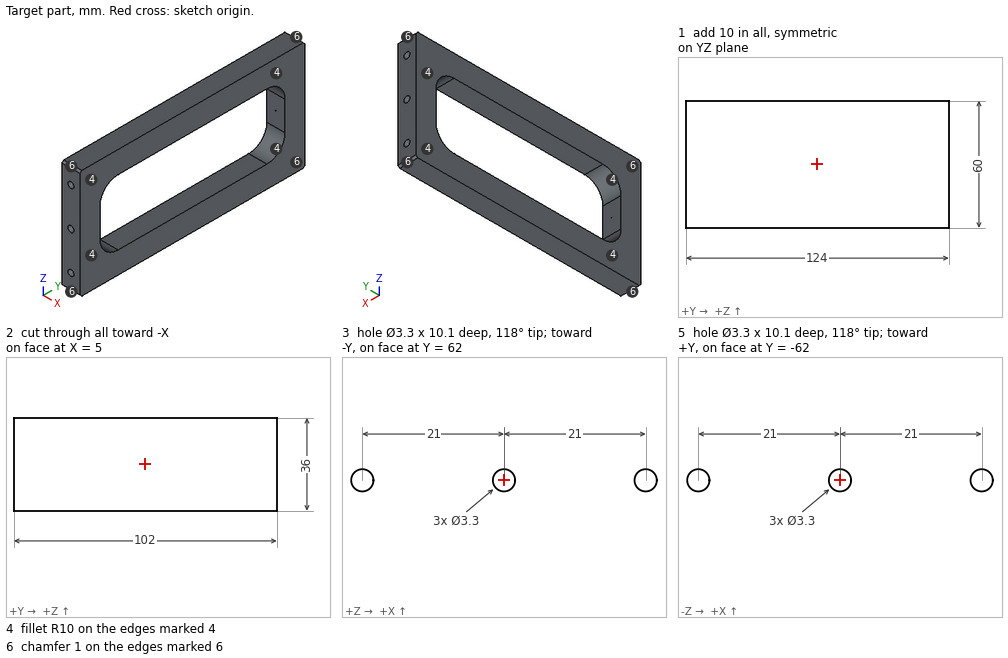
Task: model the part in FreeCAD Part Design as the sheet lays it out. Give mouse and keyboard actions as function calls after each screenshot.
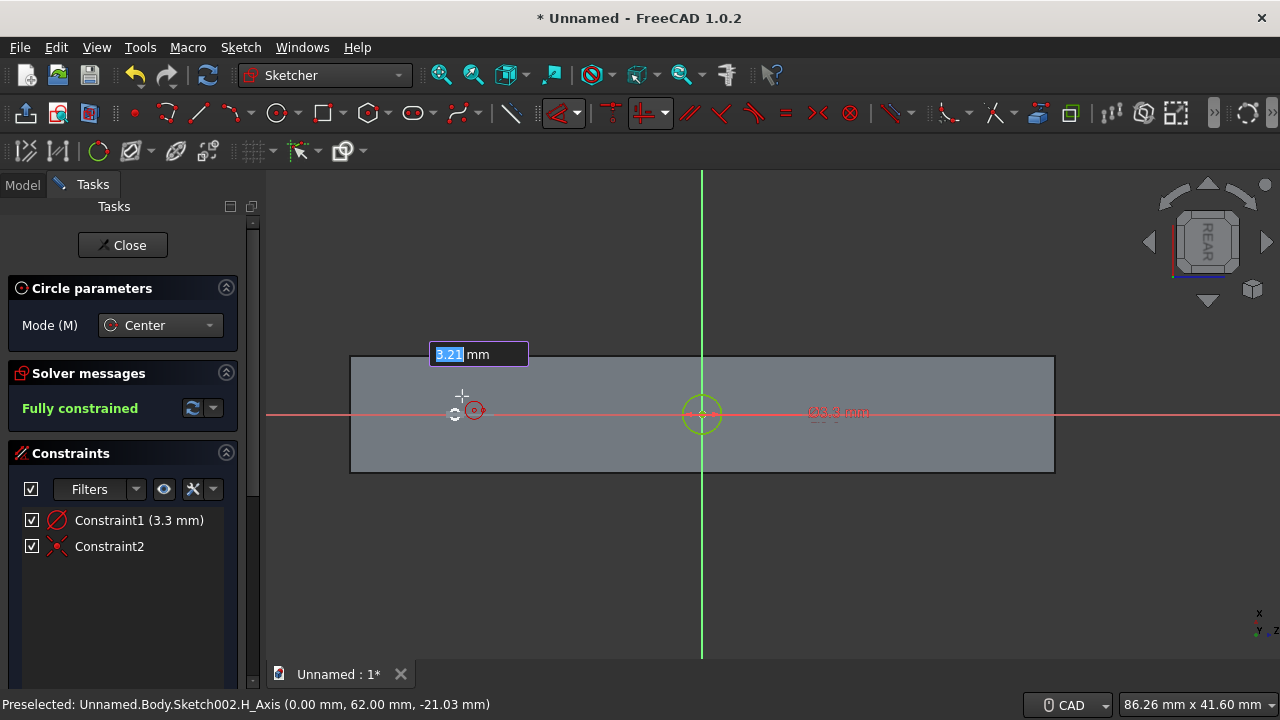
text(3.3)
key(Return)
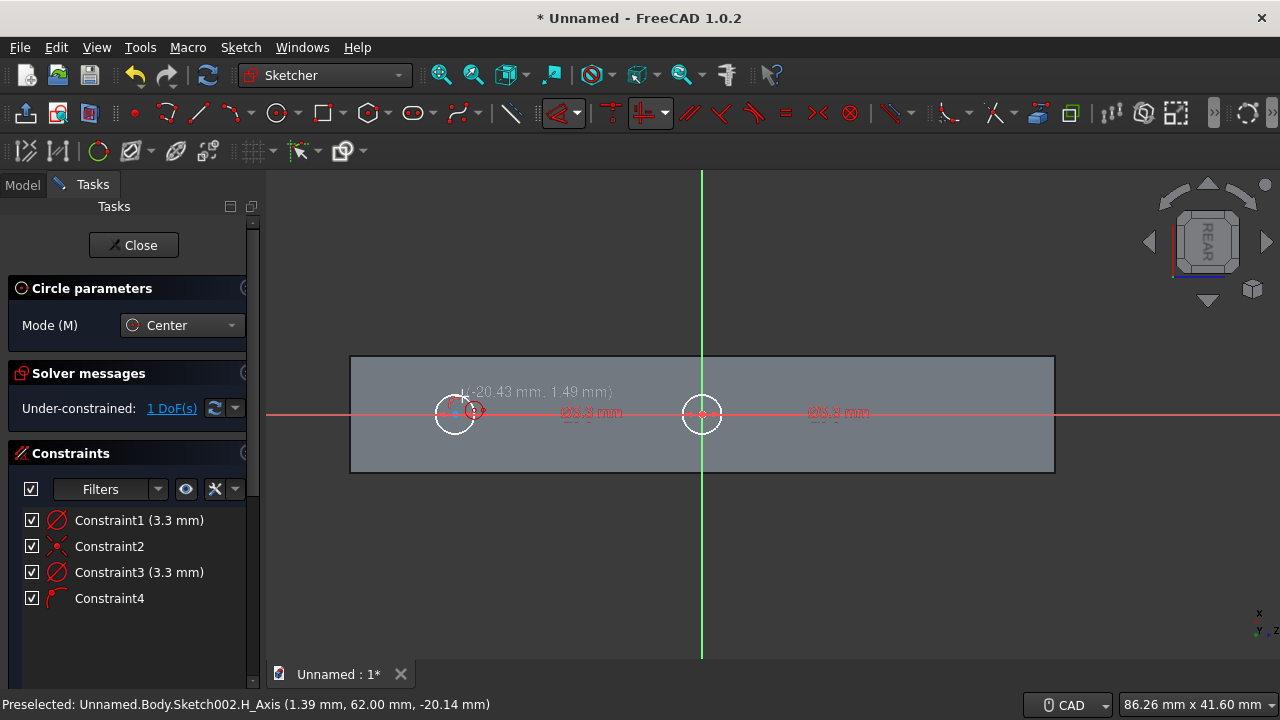
click(949, 414)
move(956, 396)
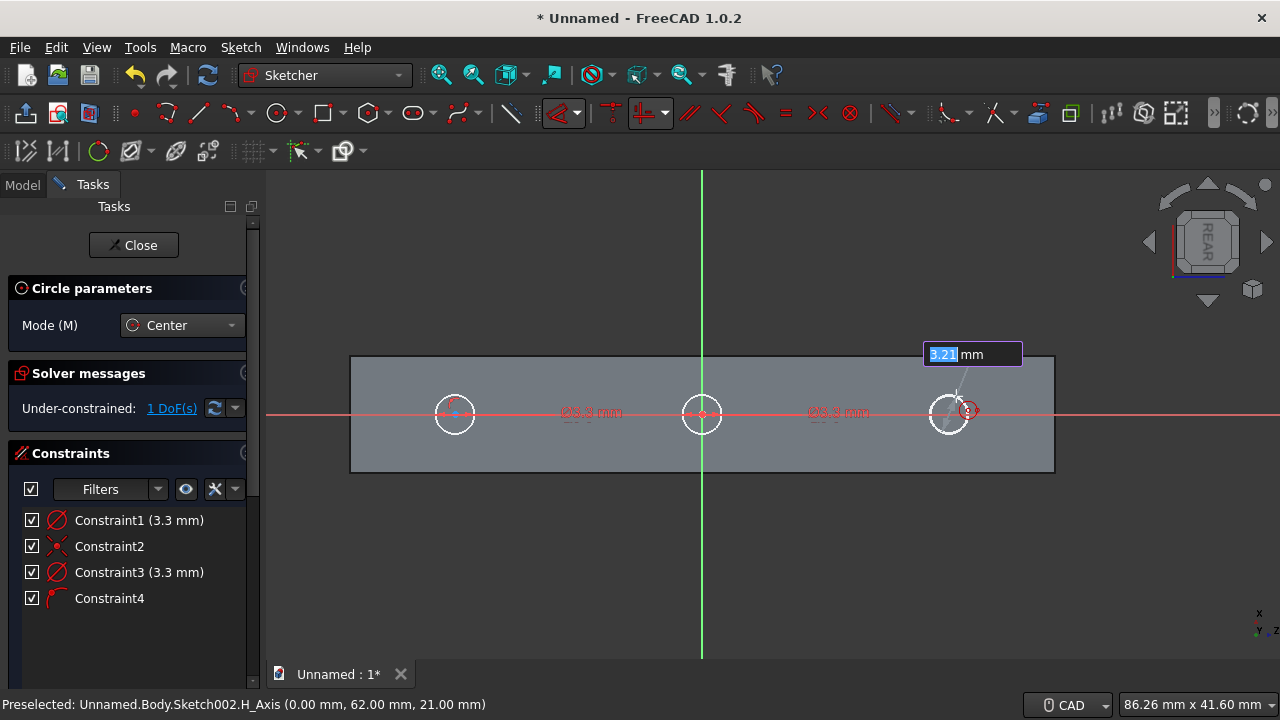
text(3.3)
key(Return)
key(Escape)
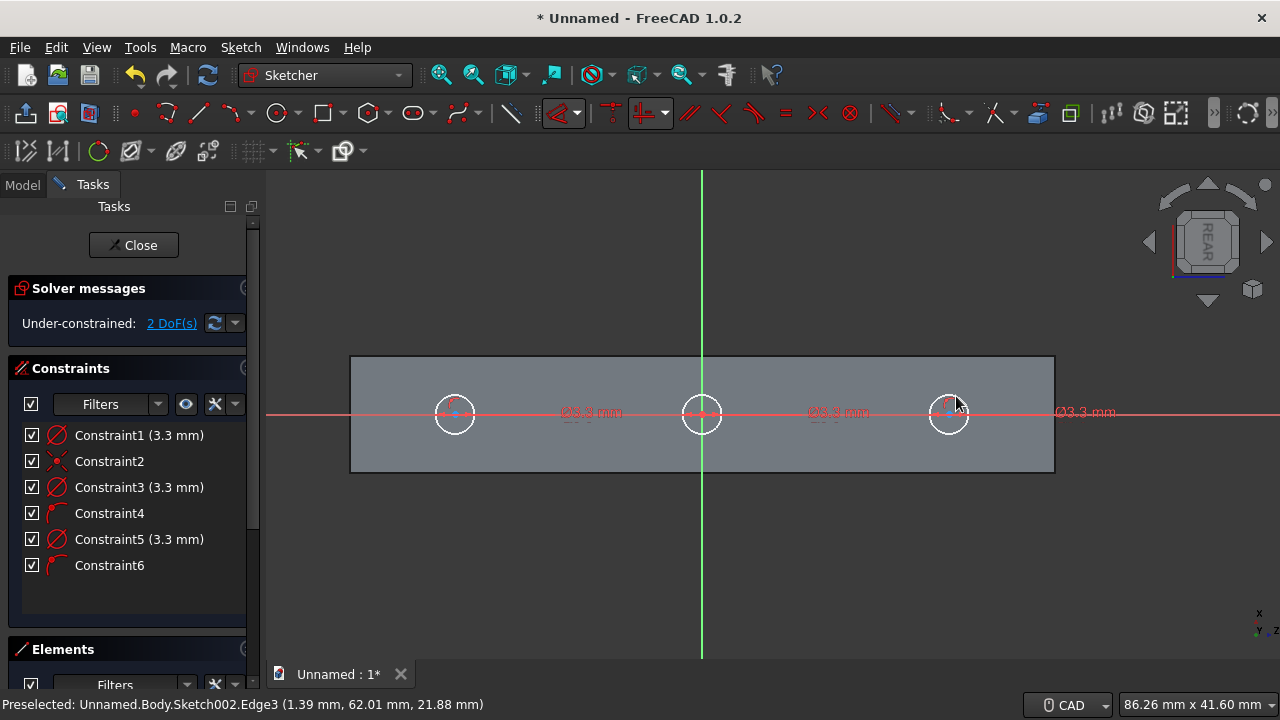
click(455, 414)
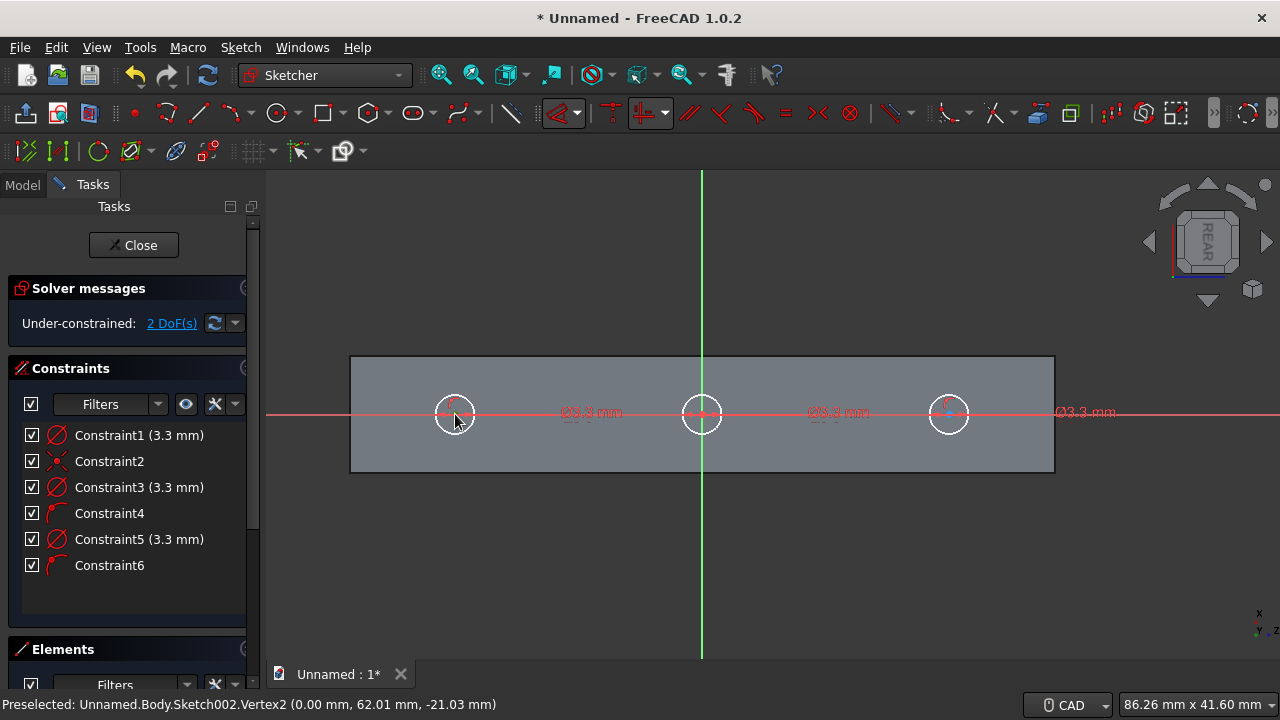
click(580, 114)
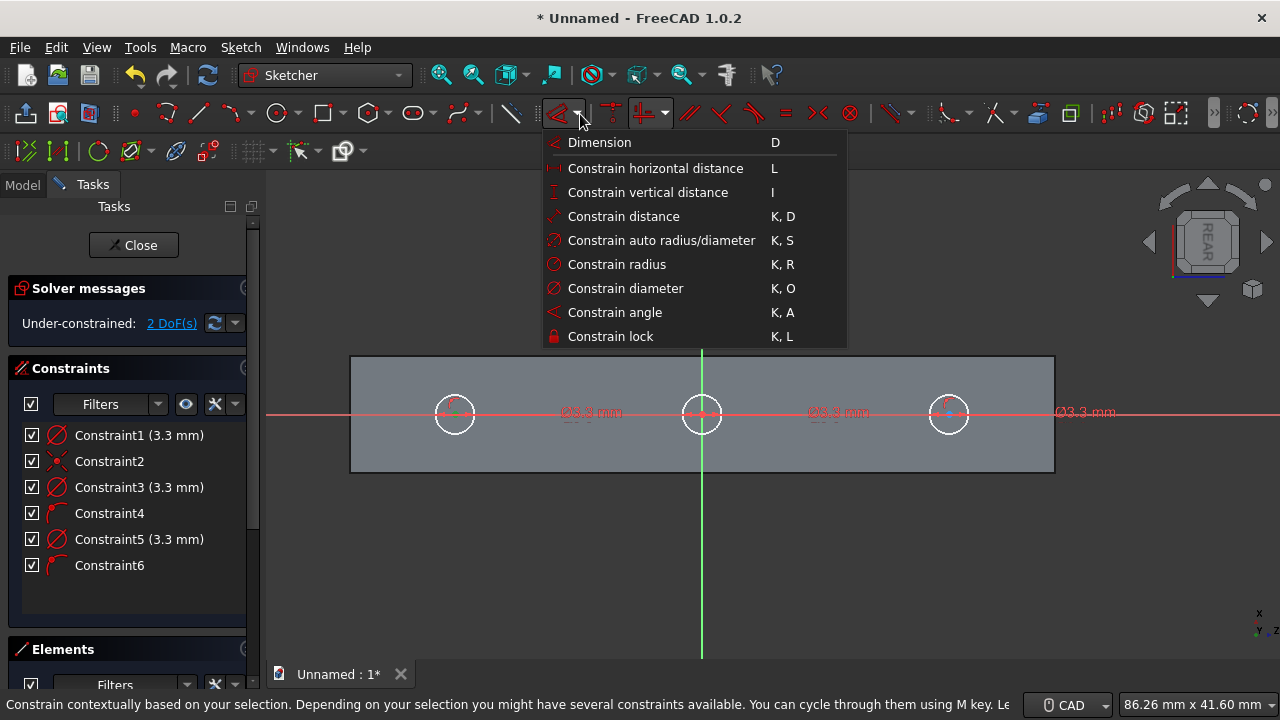
click(695, 168)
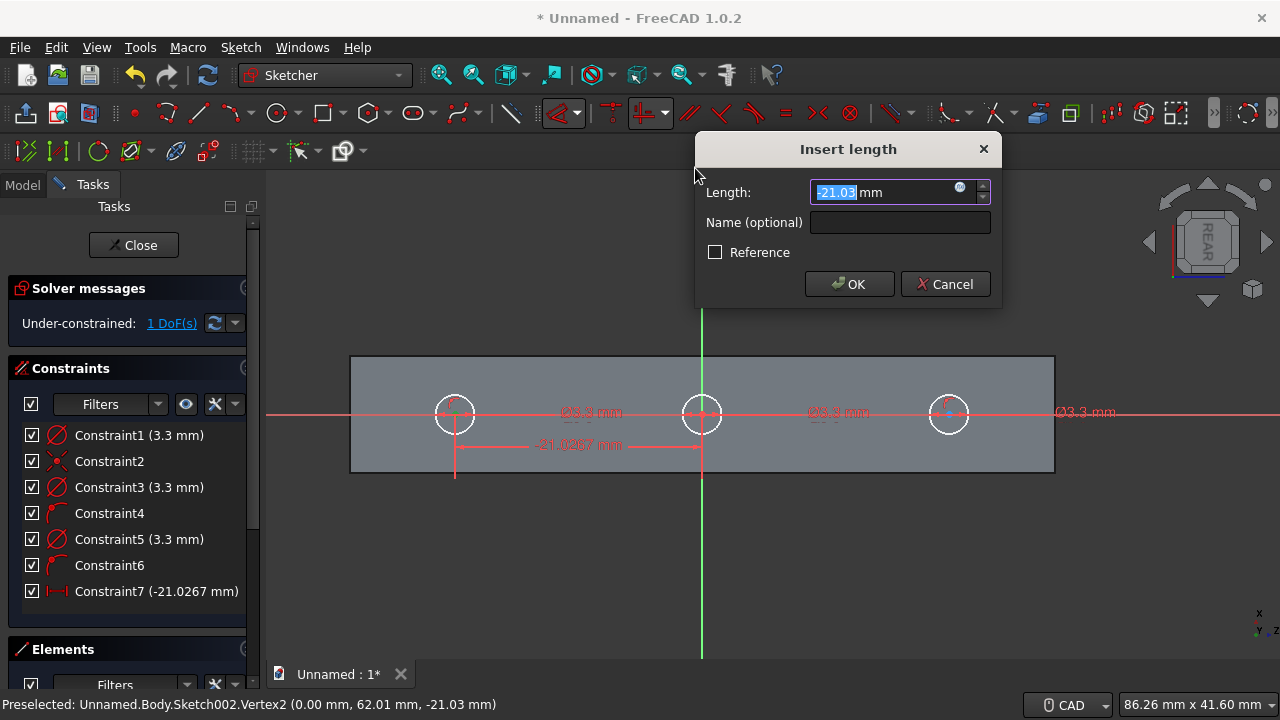
text(-21)
key(Return)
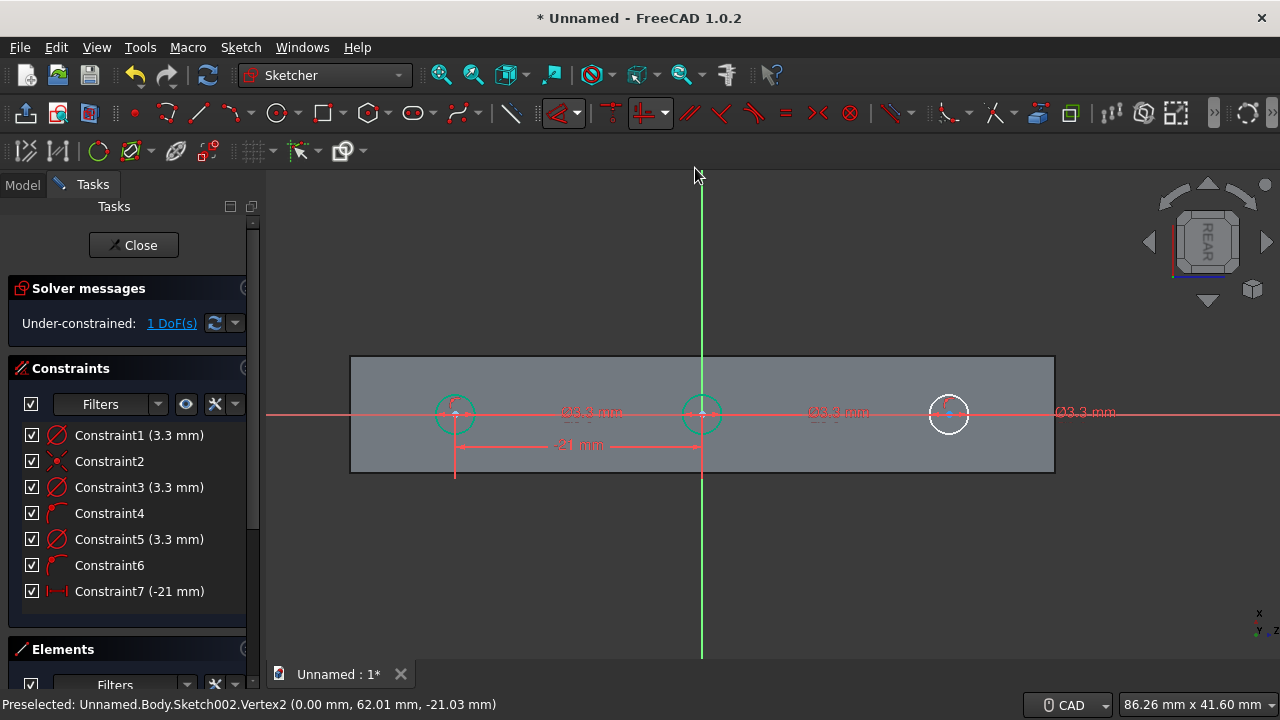
click(949, 414)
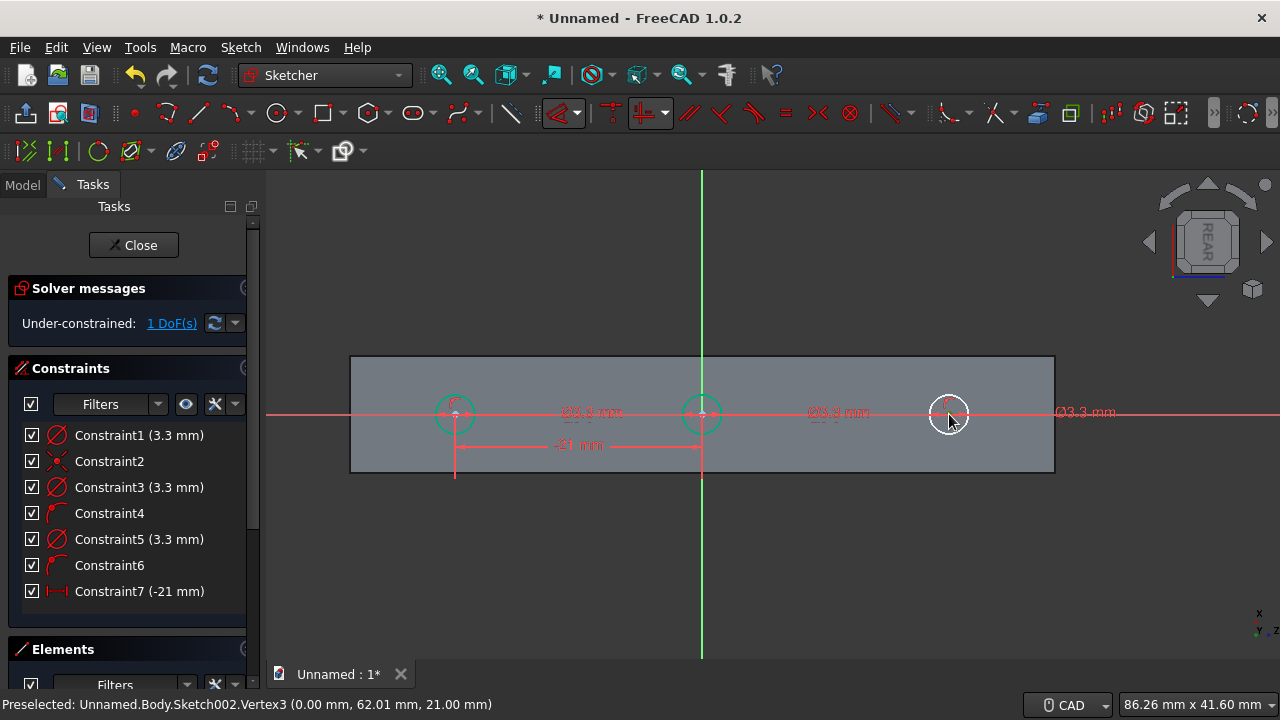
key(l)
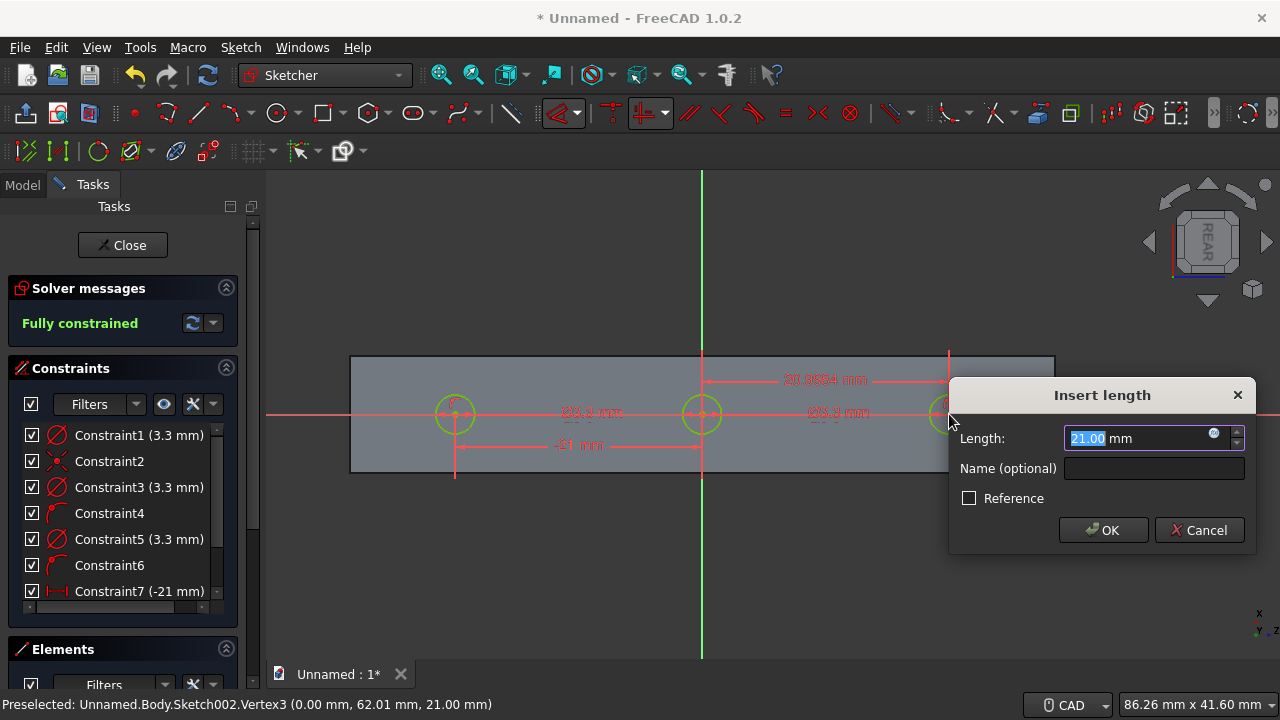
text(21)
key(Return)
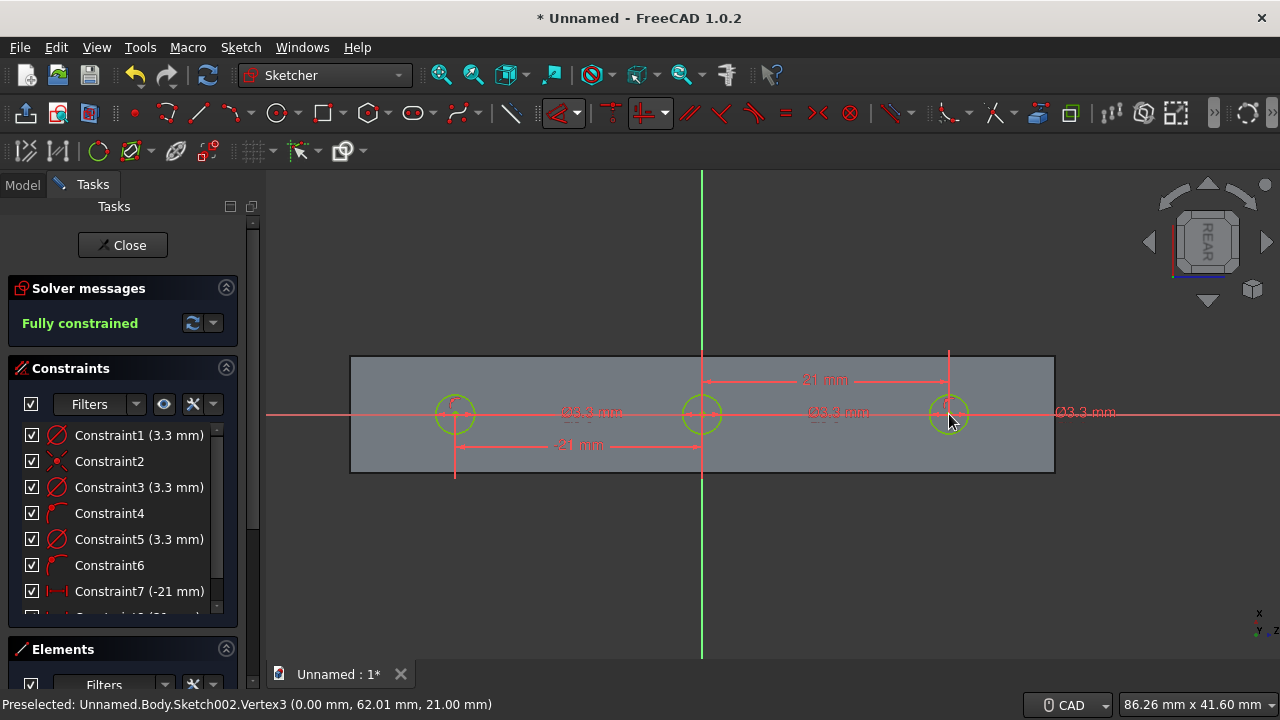
click(123, 245)